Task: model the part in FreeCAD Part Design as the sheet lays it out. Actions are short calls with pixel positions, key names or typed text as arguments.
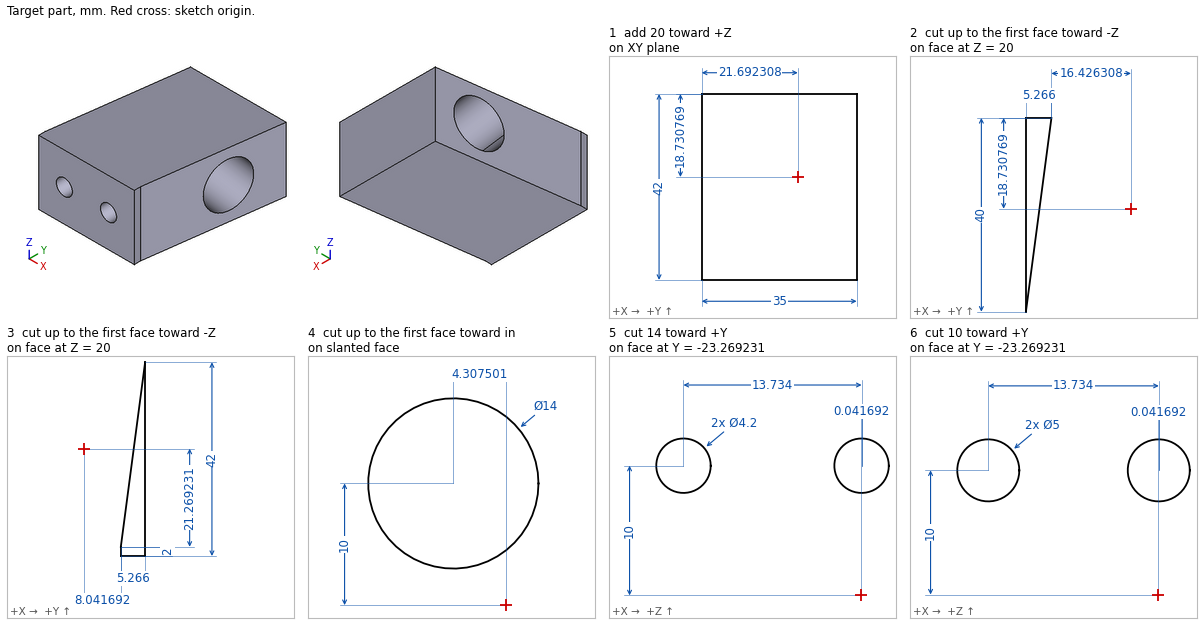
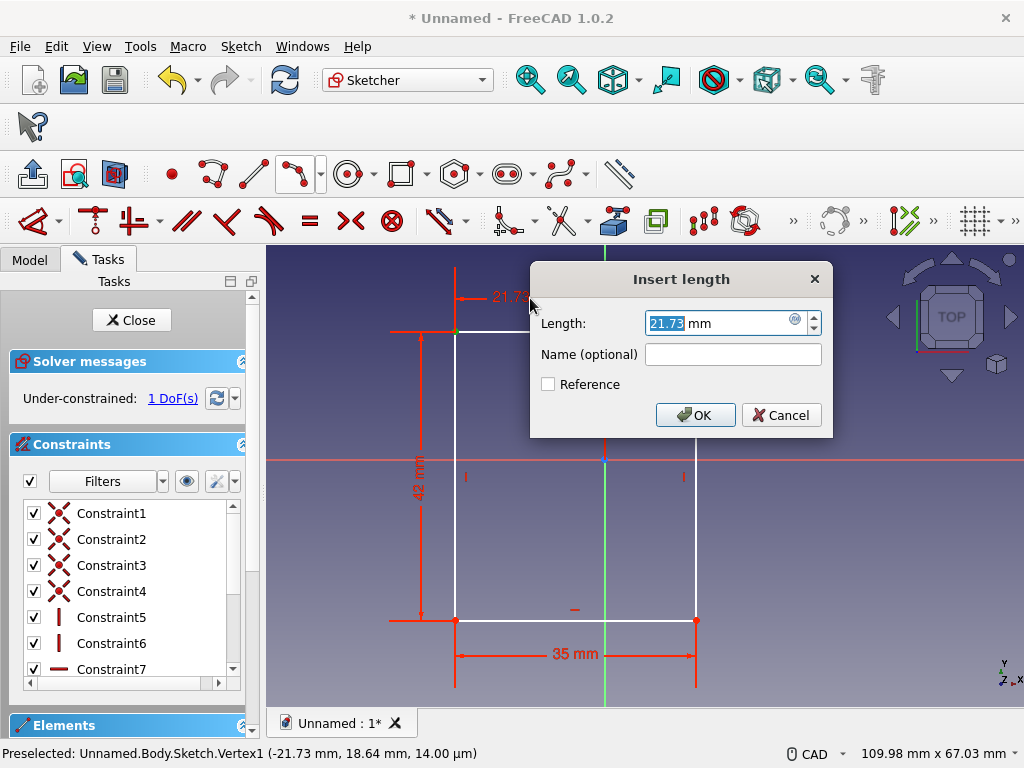
text(21.692308)
key(Return)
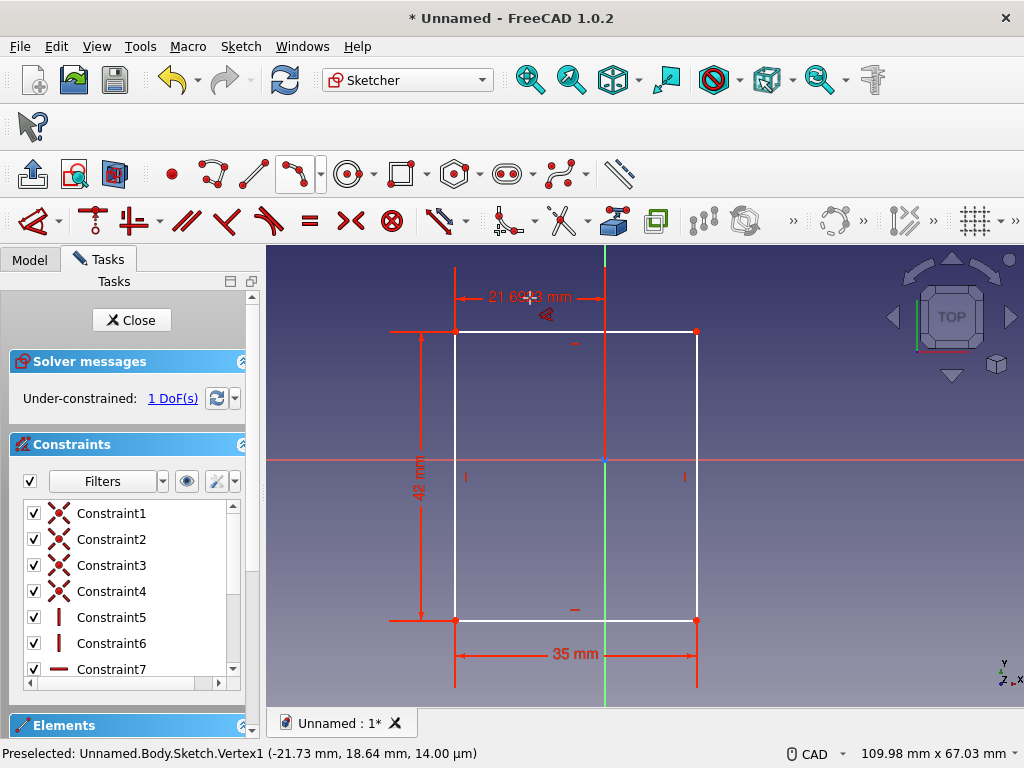
click(455, 332)
click(421, 396)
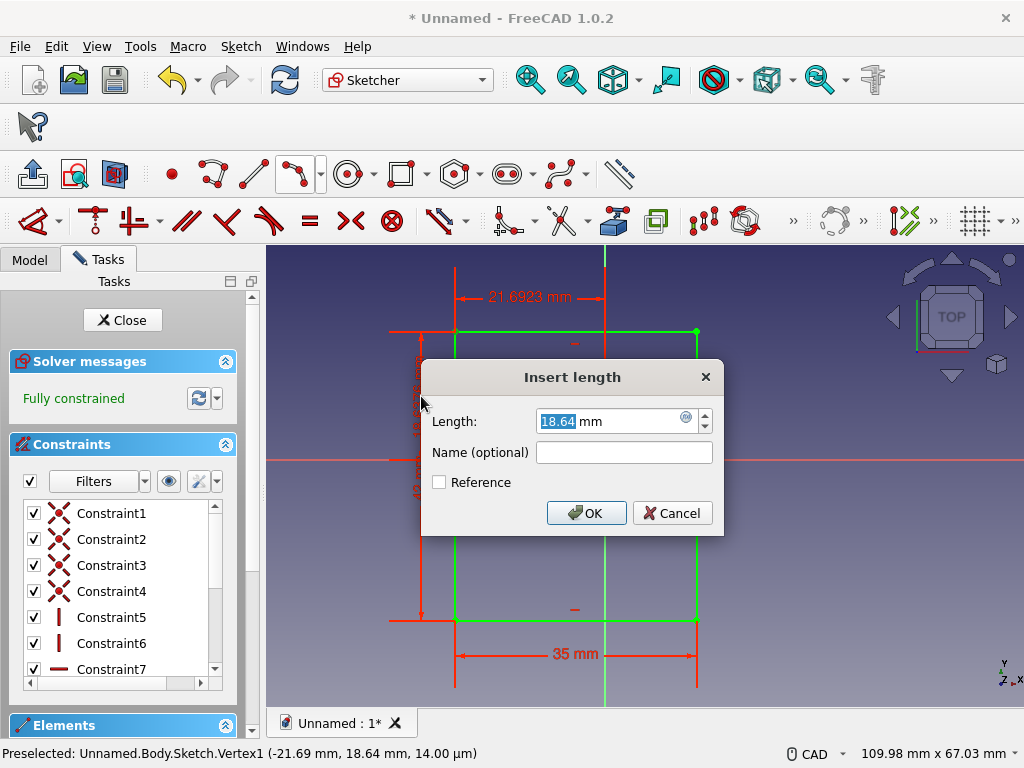
text(18.730769)
key(Return)
key(Escape)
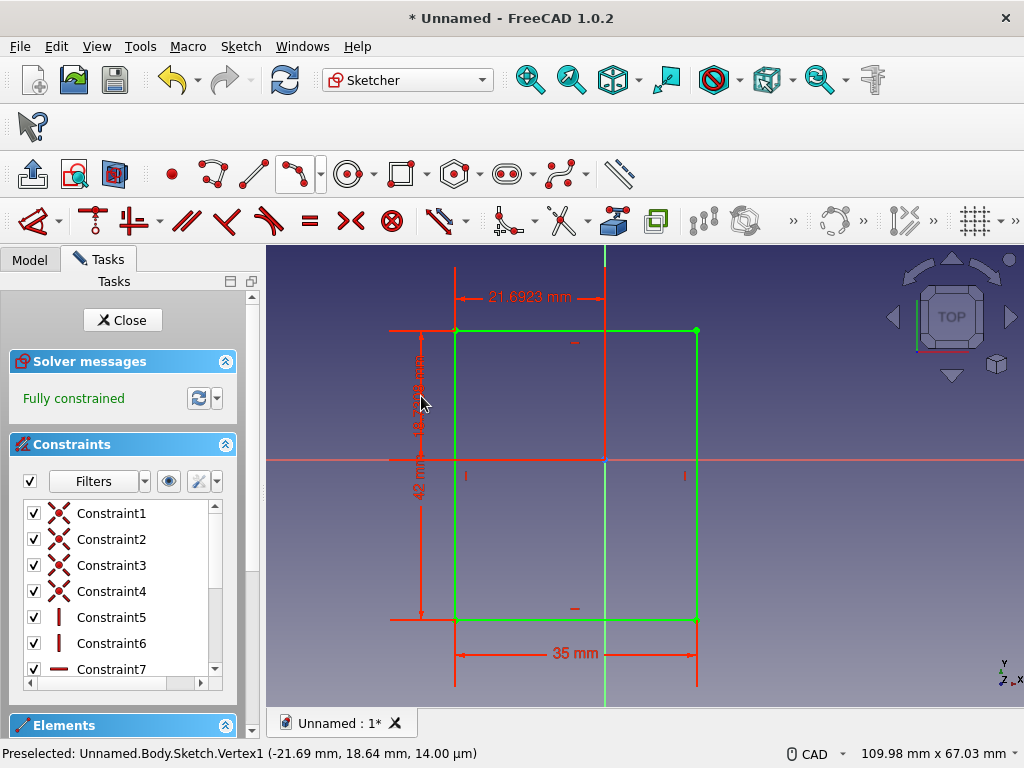
click(123, 320)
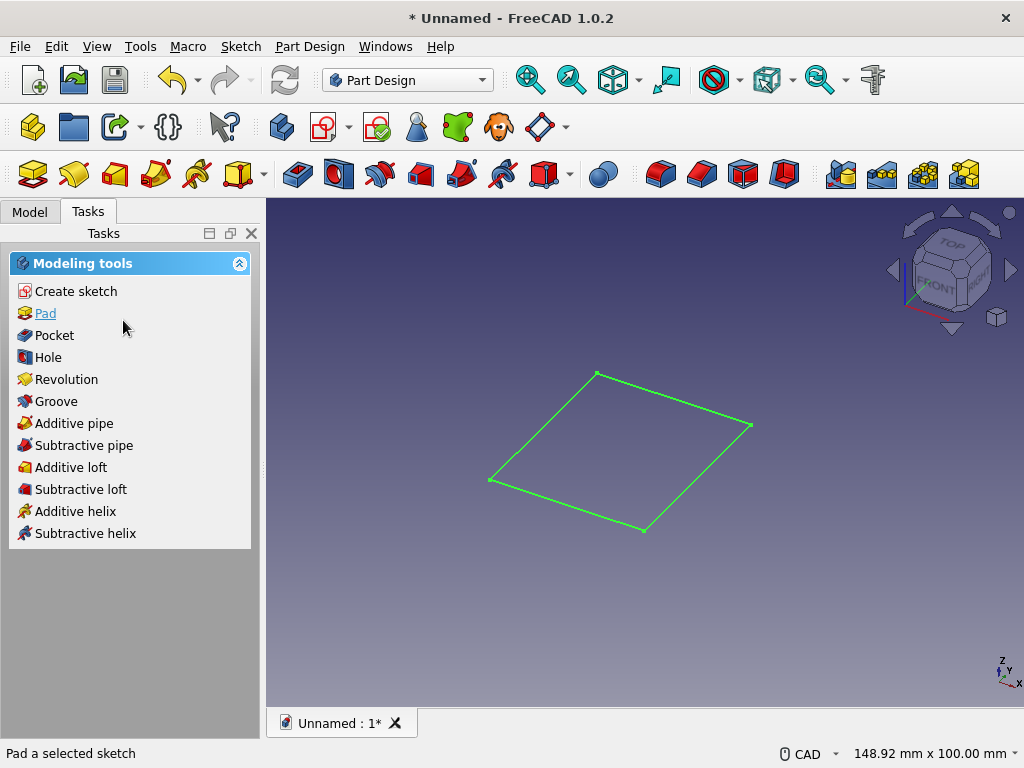
click(33, 174)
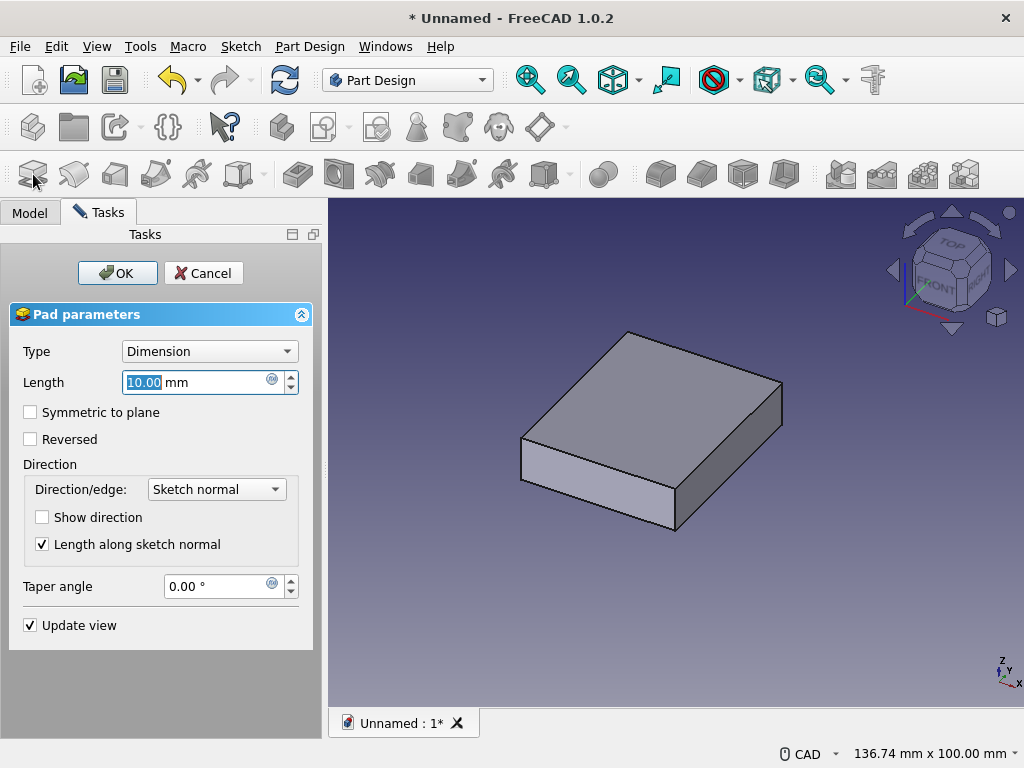
text(20)
key(Tab)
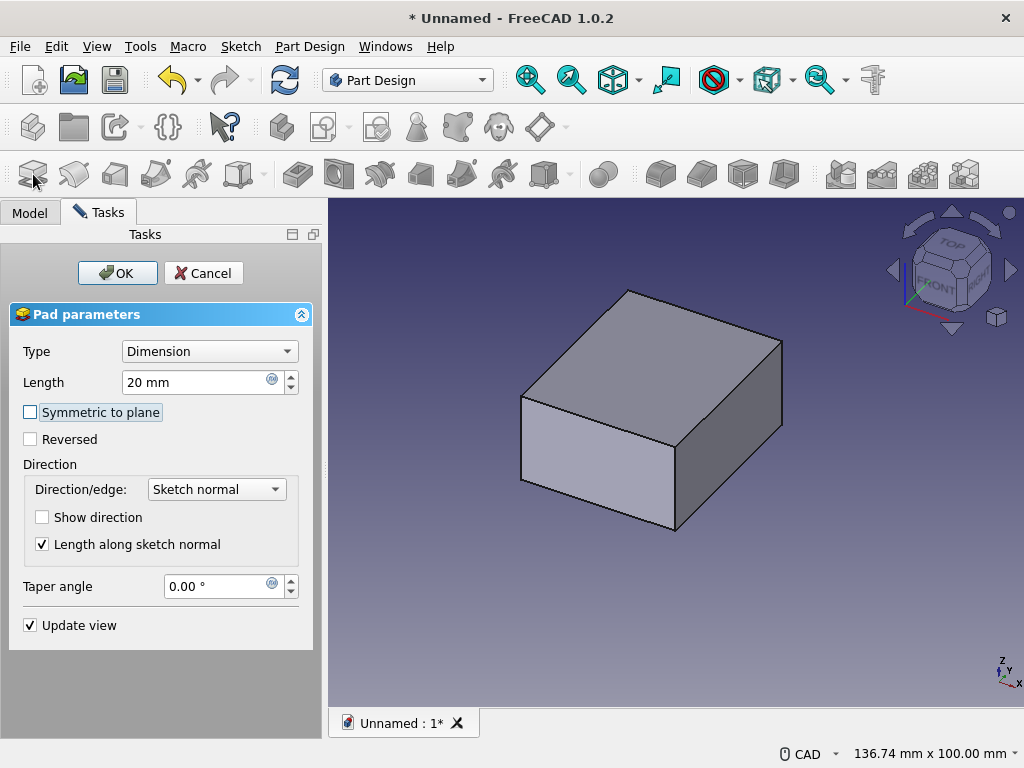
click(118, 273)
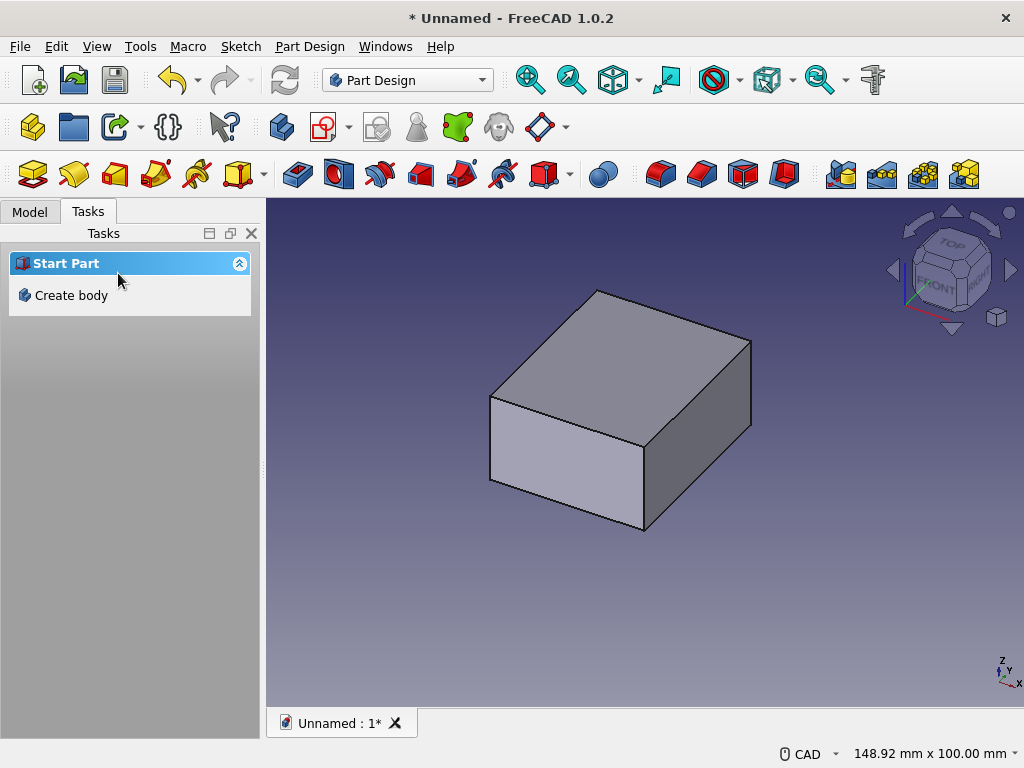
click(621, 368)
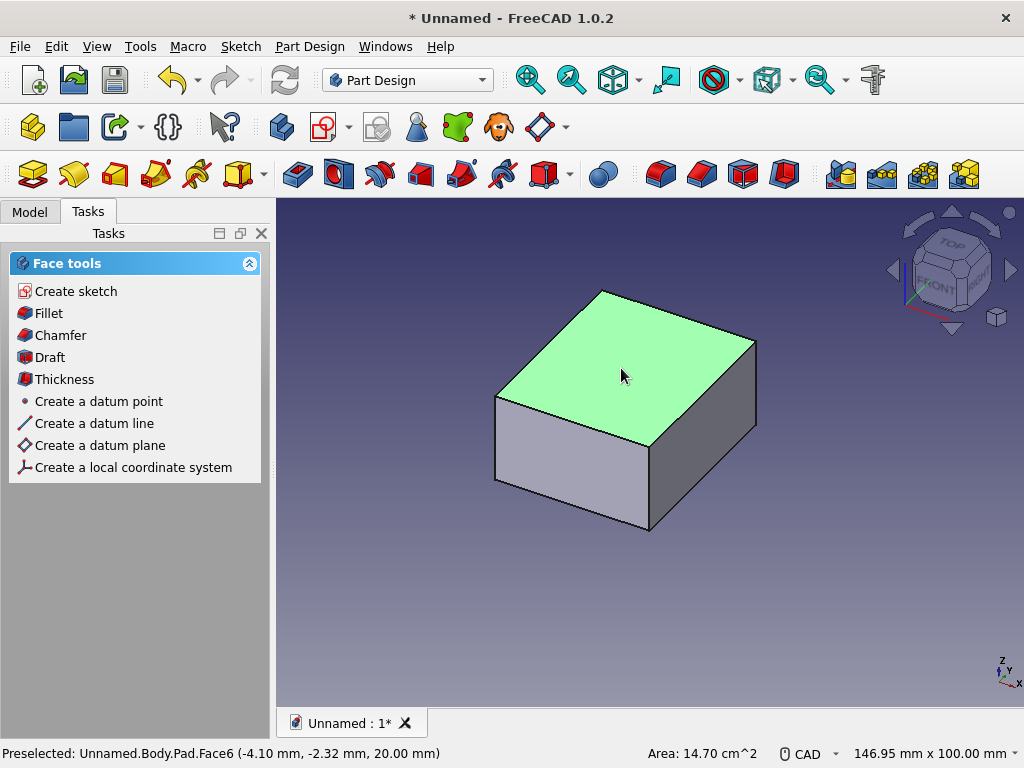
click(322, 128)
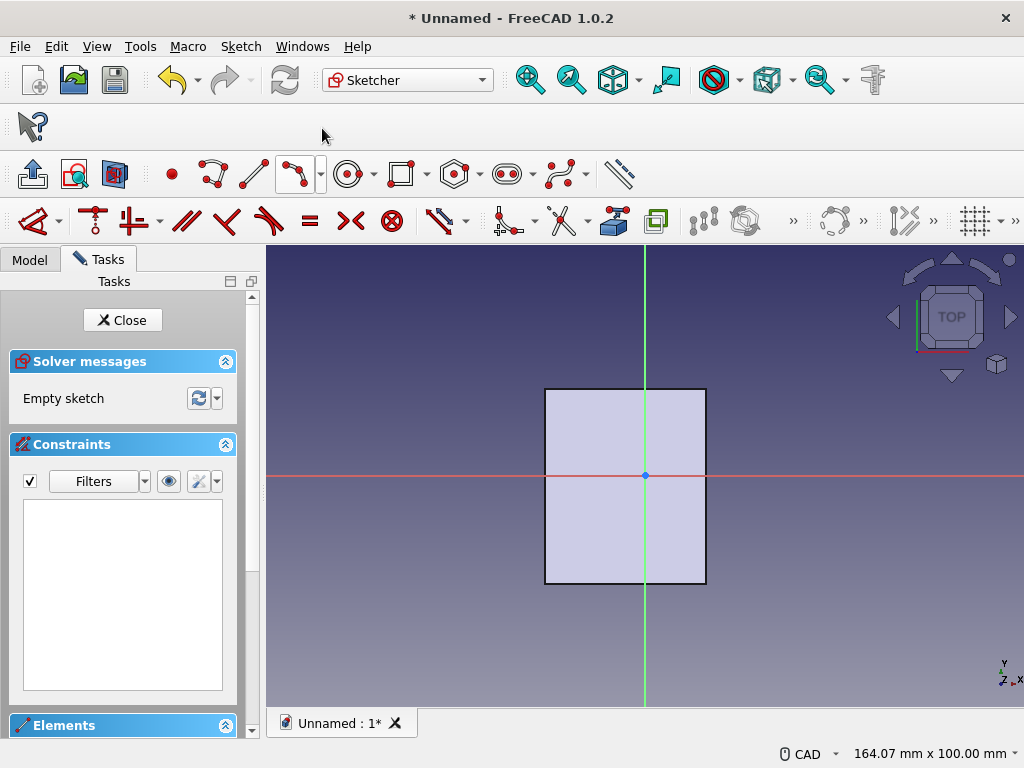
scroll(632, 494, up, 2)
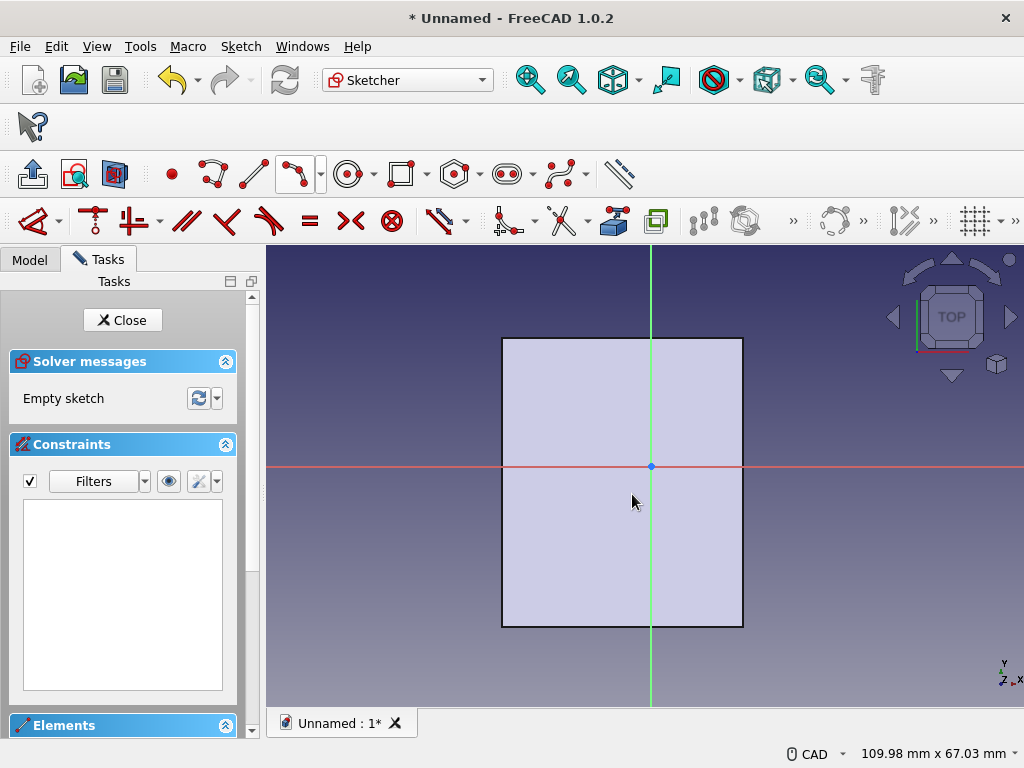
click(213, 174)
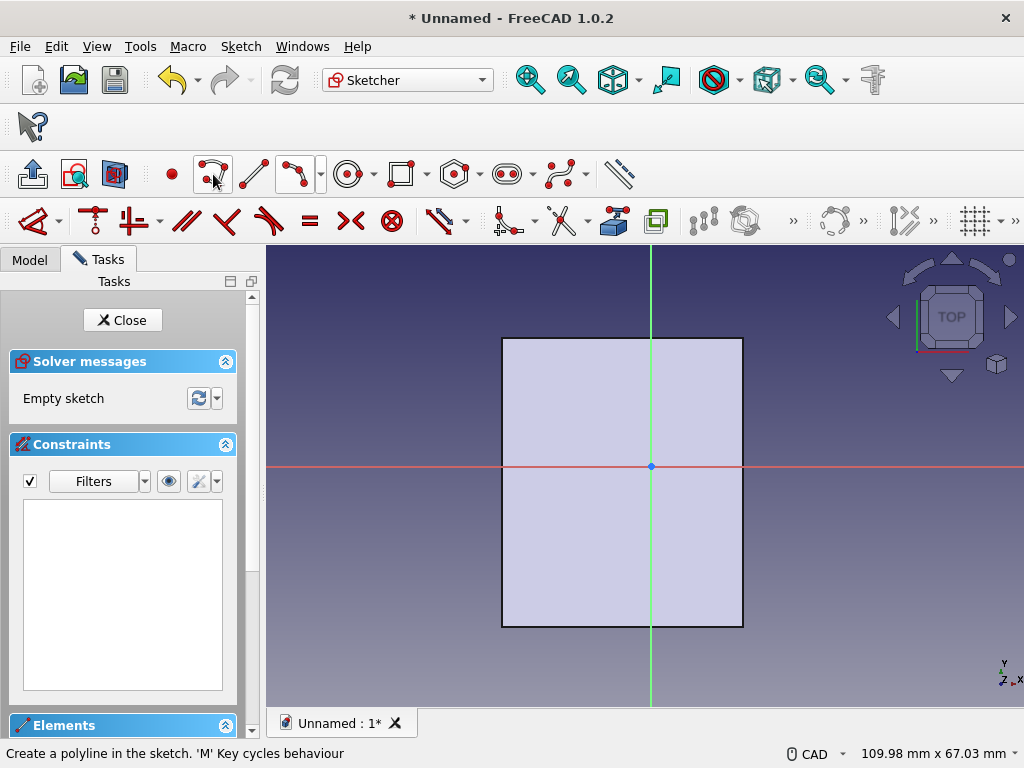
click(538, 338)
click(502, 338)
click(502, 613)
click(538, 339)
key(Escape)
key(Escape)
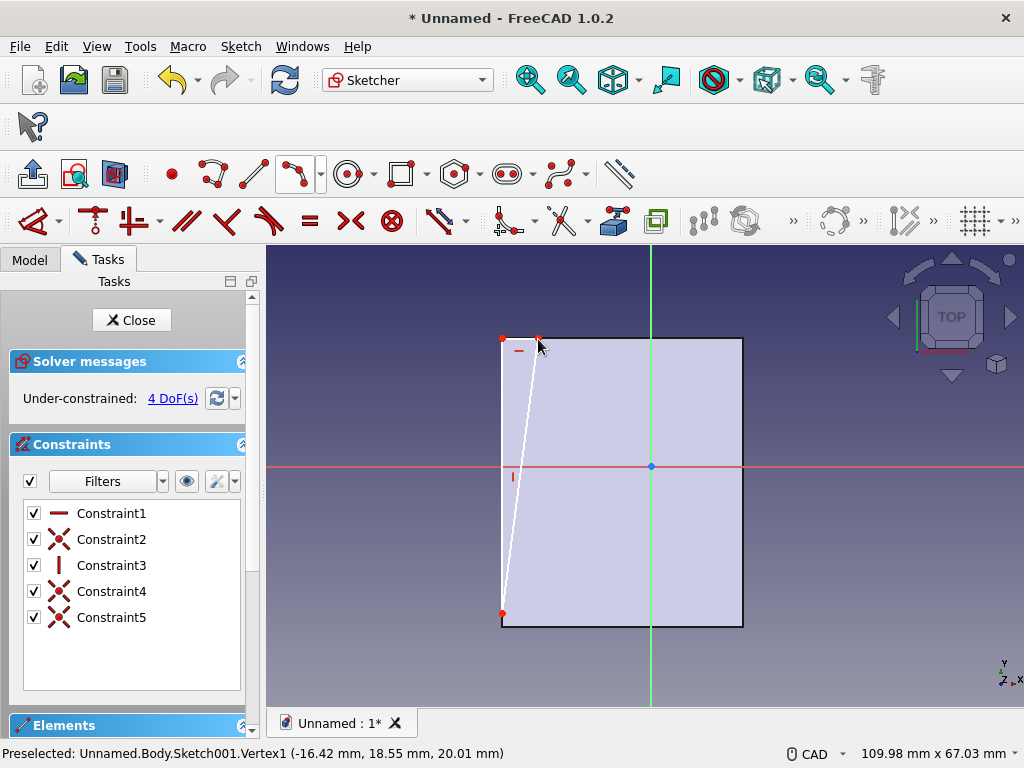
click(32, 222)